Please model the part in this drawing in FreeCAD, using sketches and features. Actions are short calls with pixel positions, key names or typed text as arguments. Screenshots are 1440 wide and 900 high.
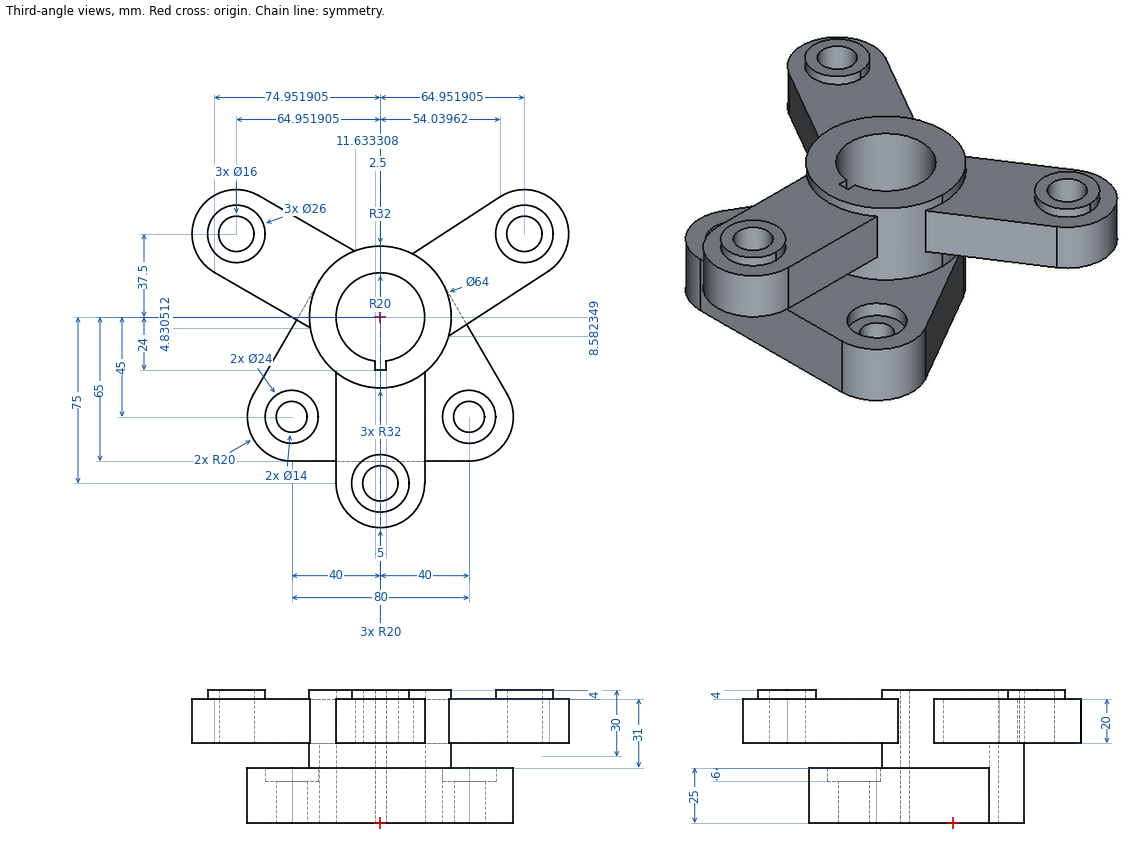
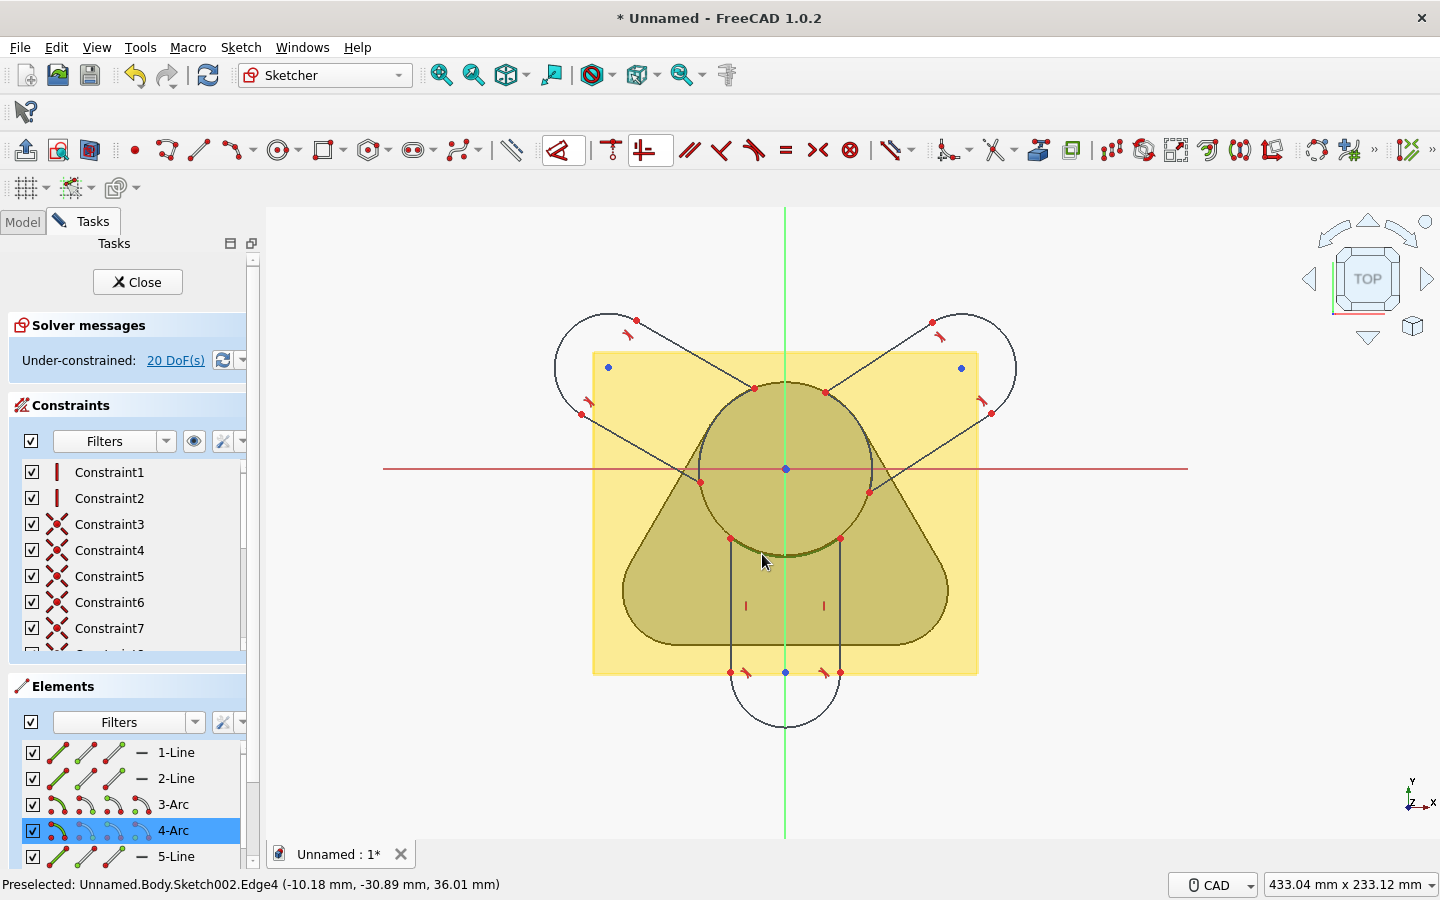
scroll(871, 458, up, 2)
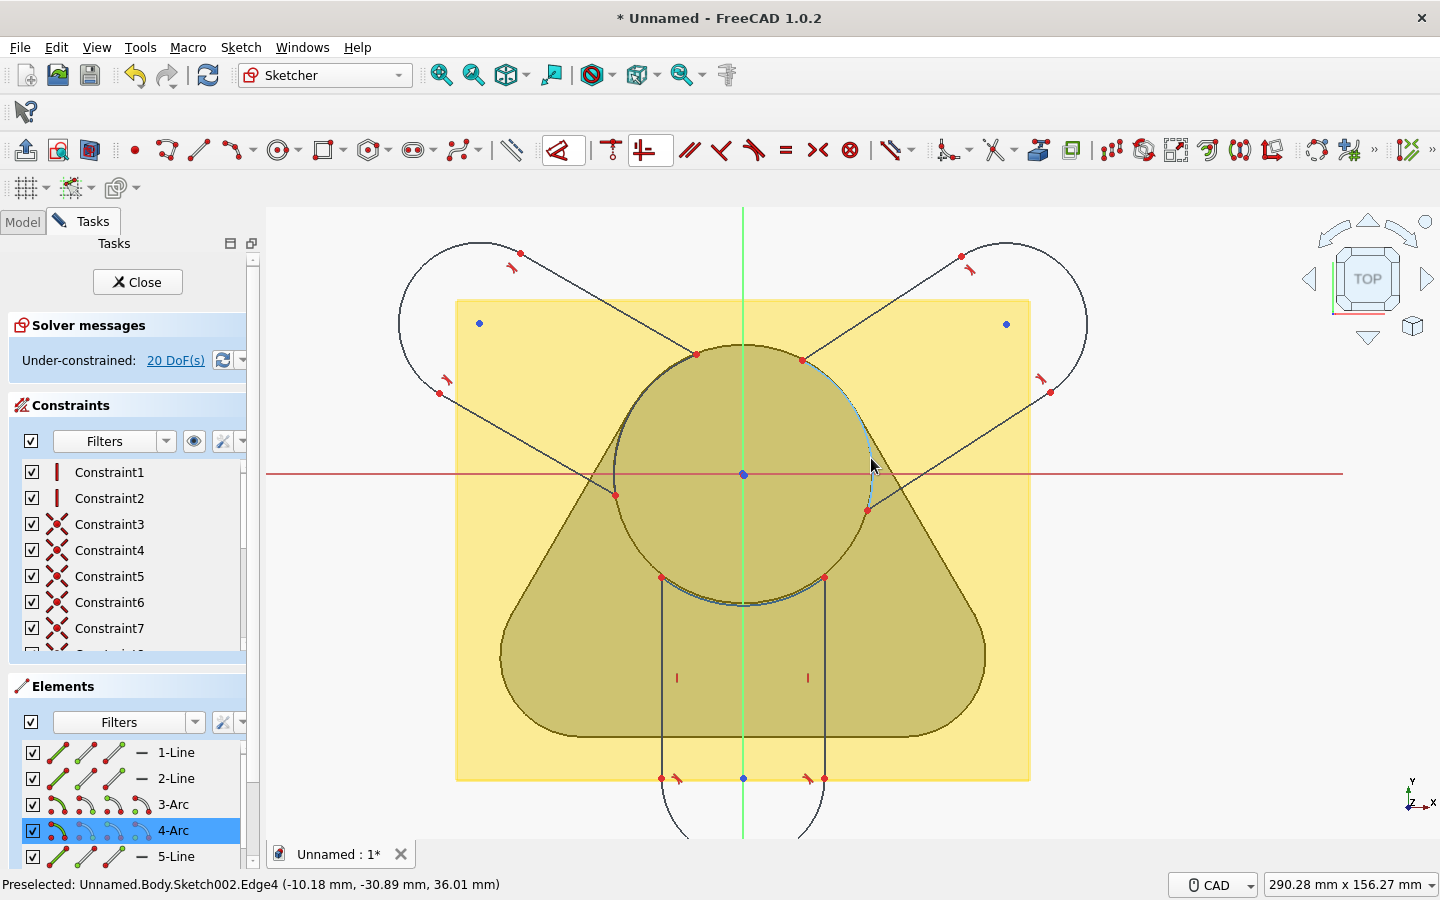
click(871, 457)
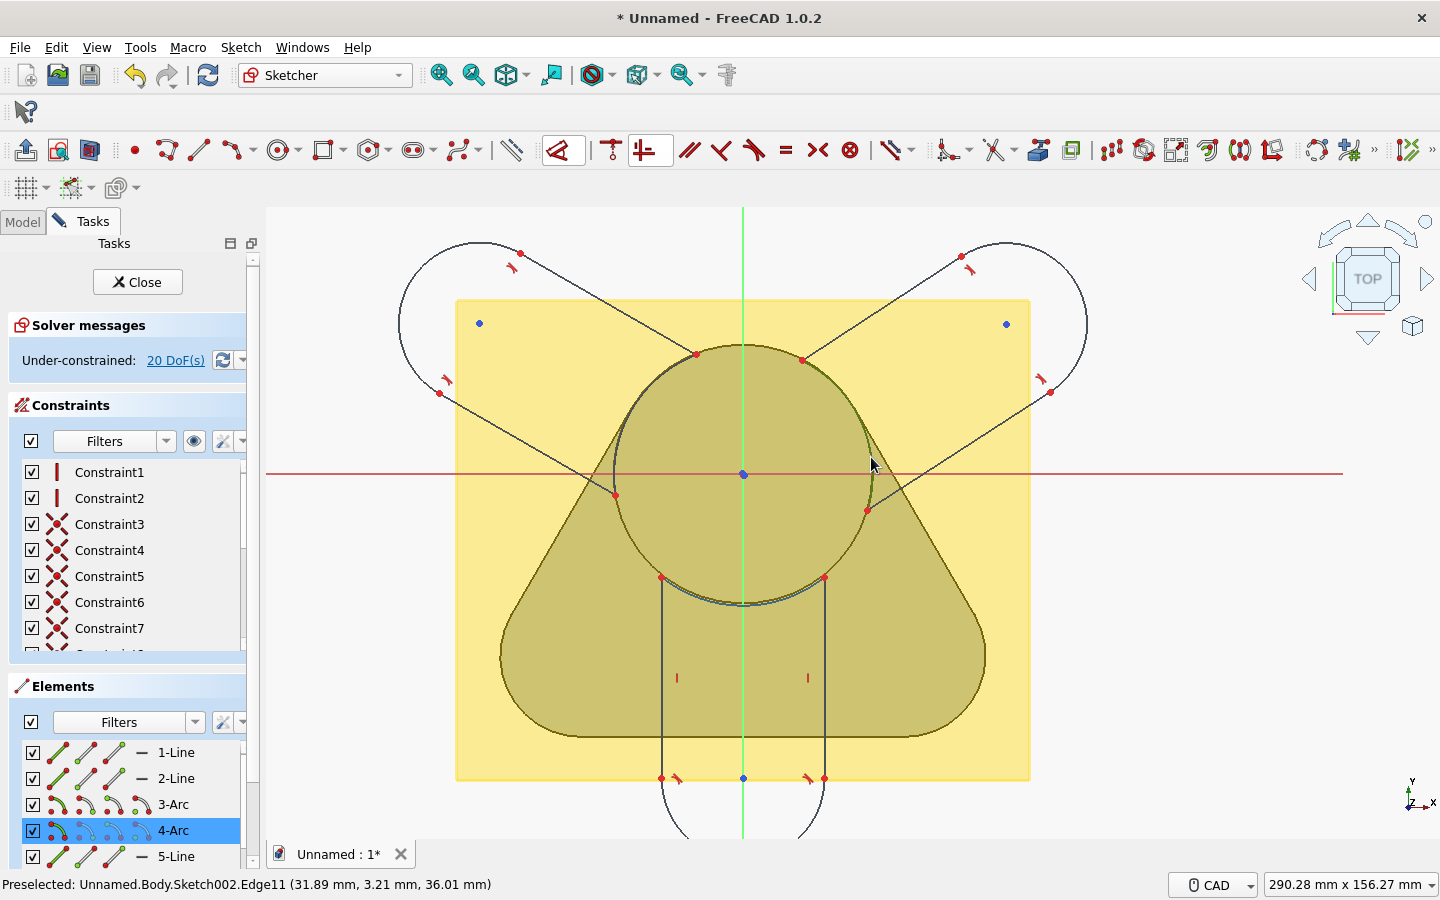
key(c)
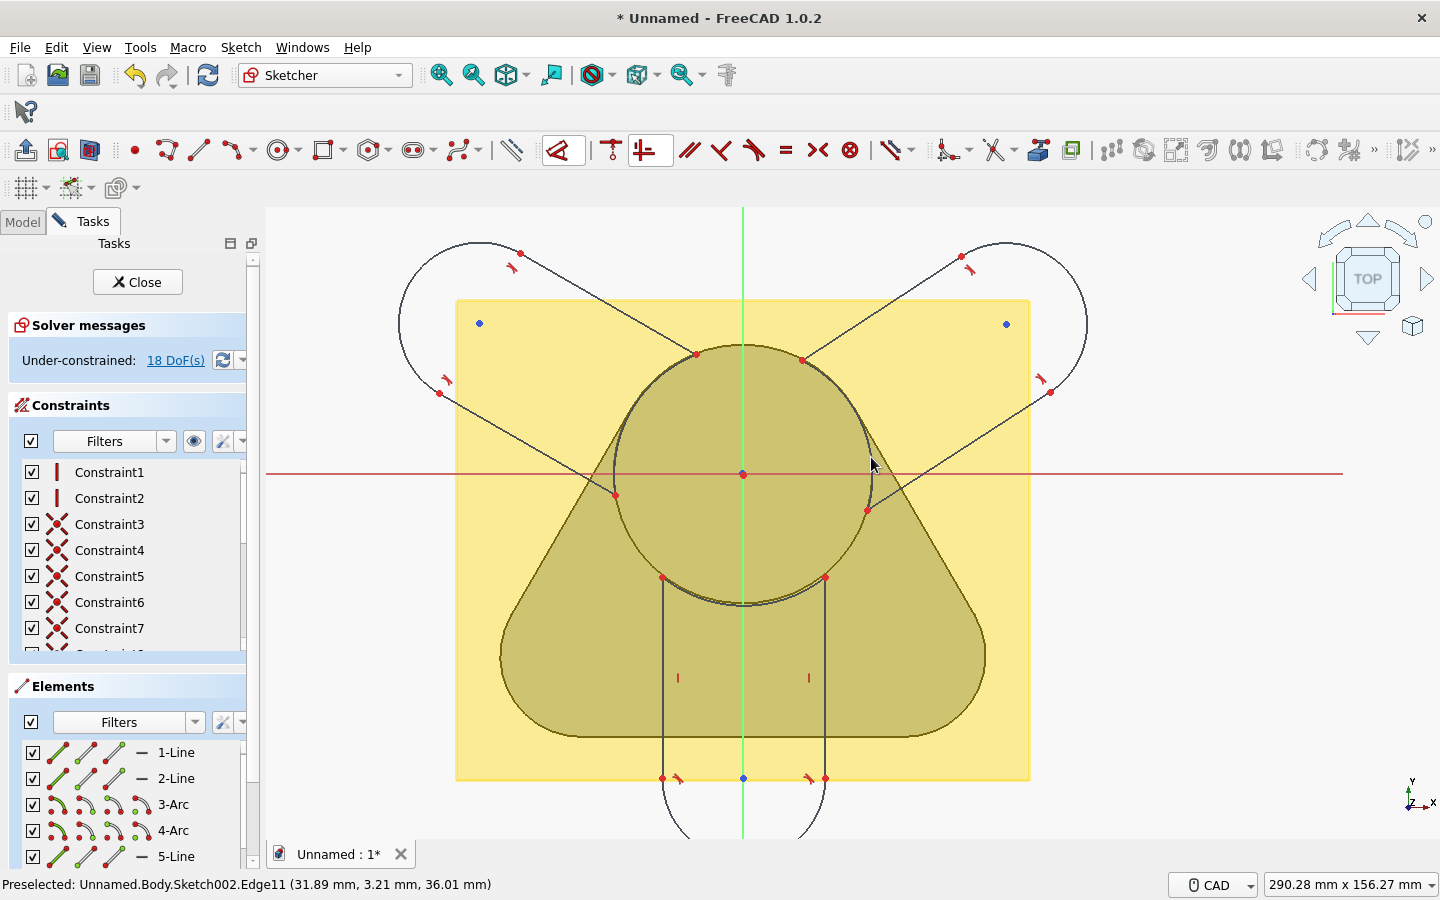
drag(733, 464, 754, 485)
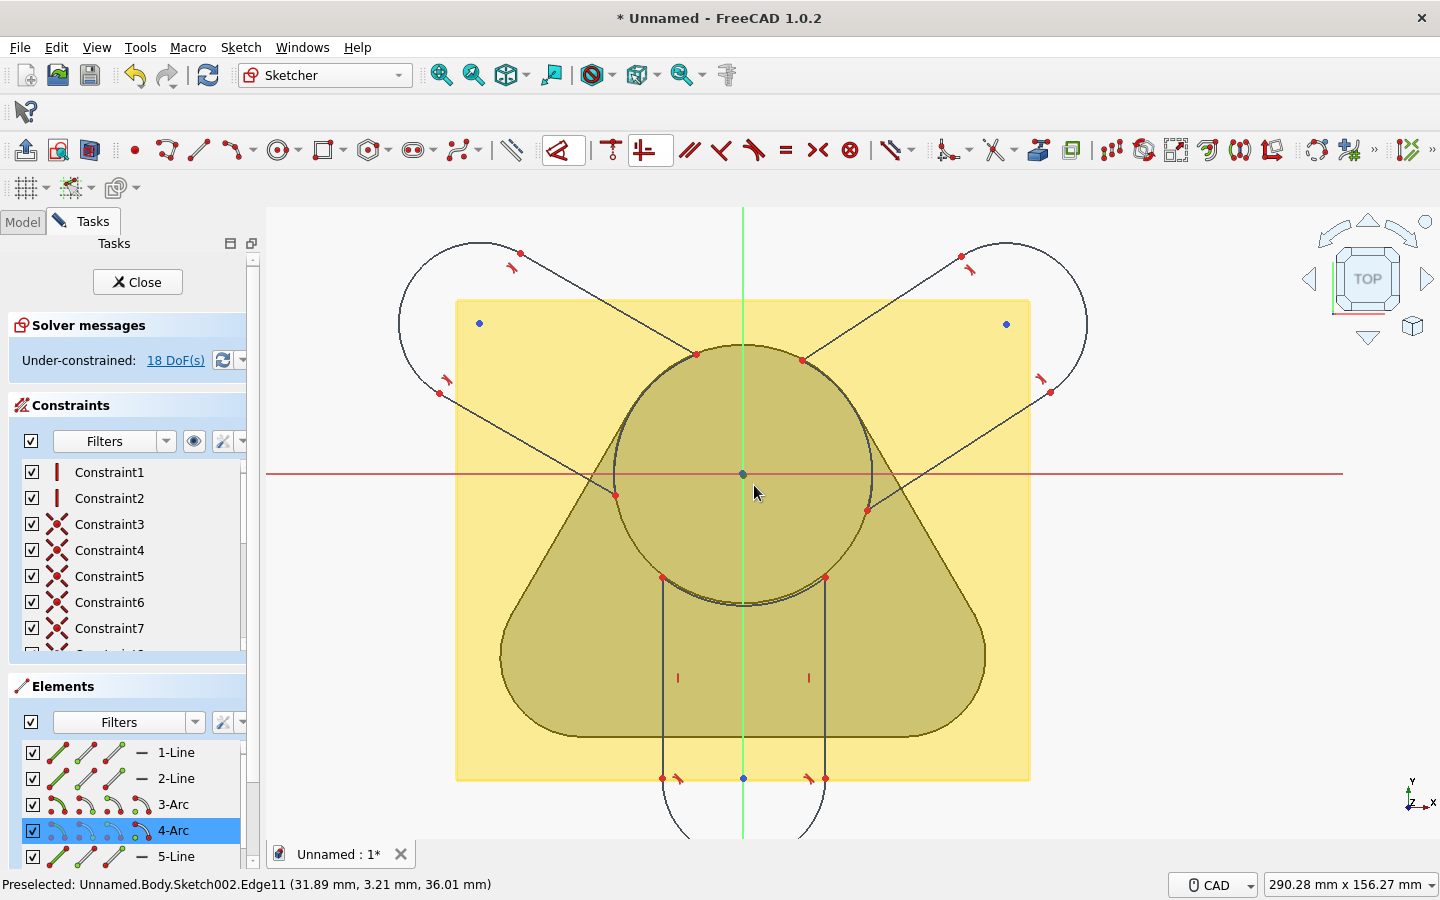
click(612, 150)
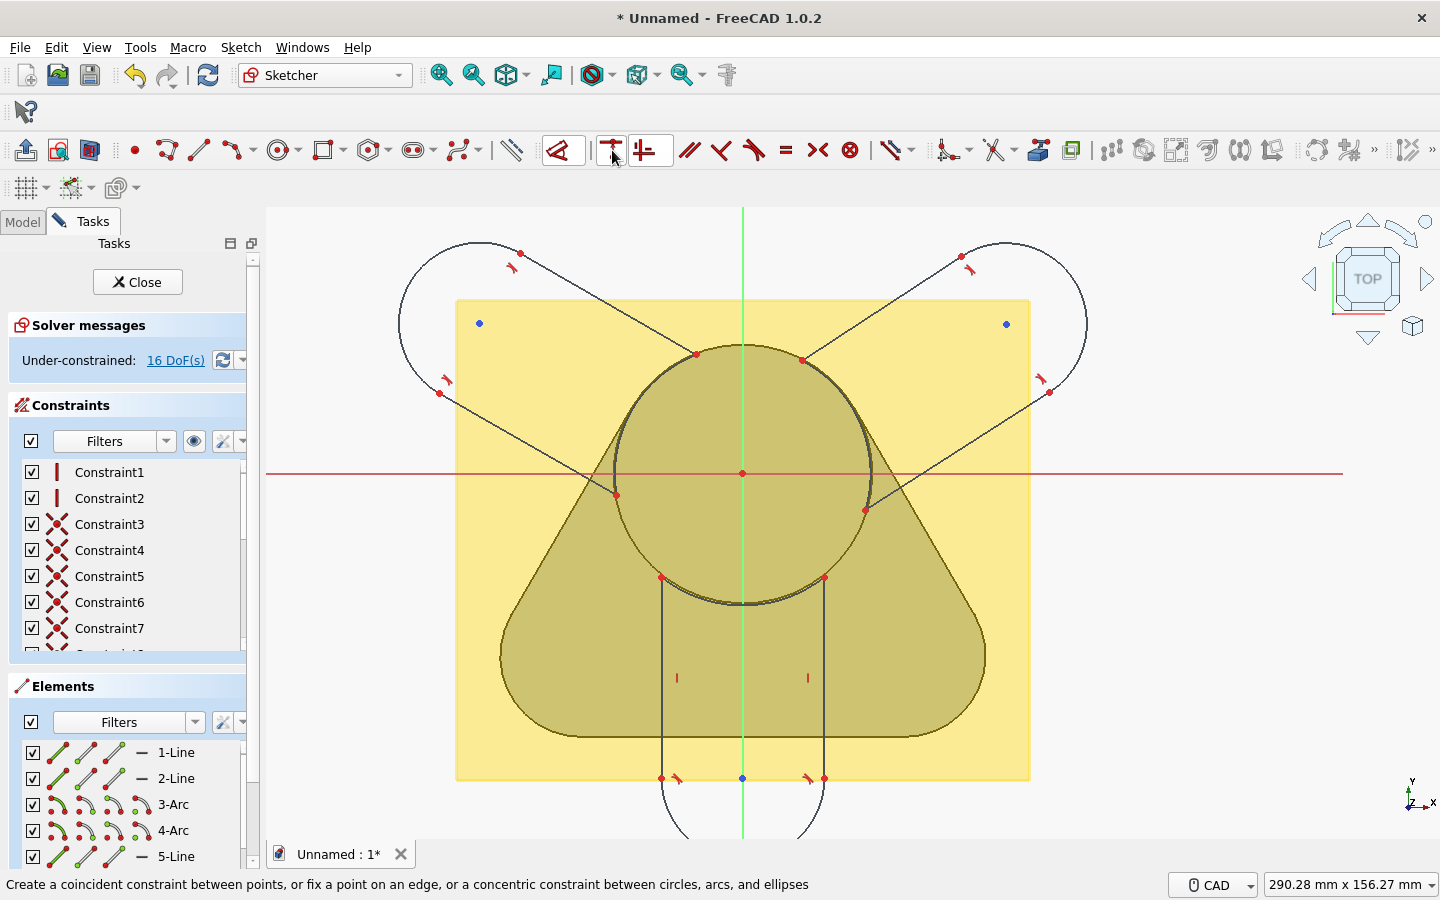
click(708, 601)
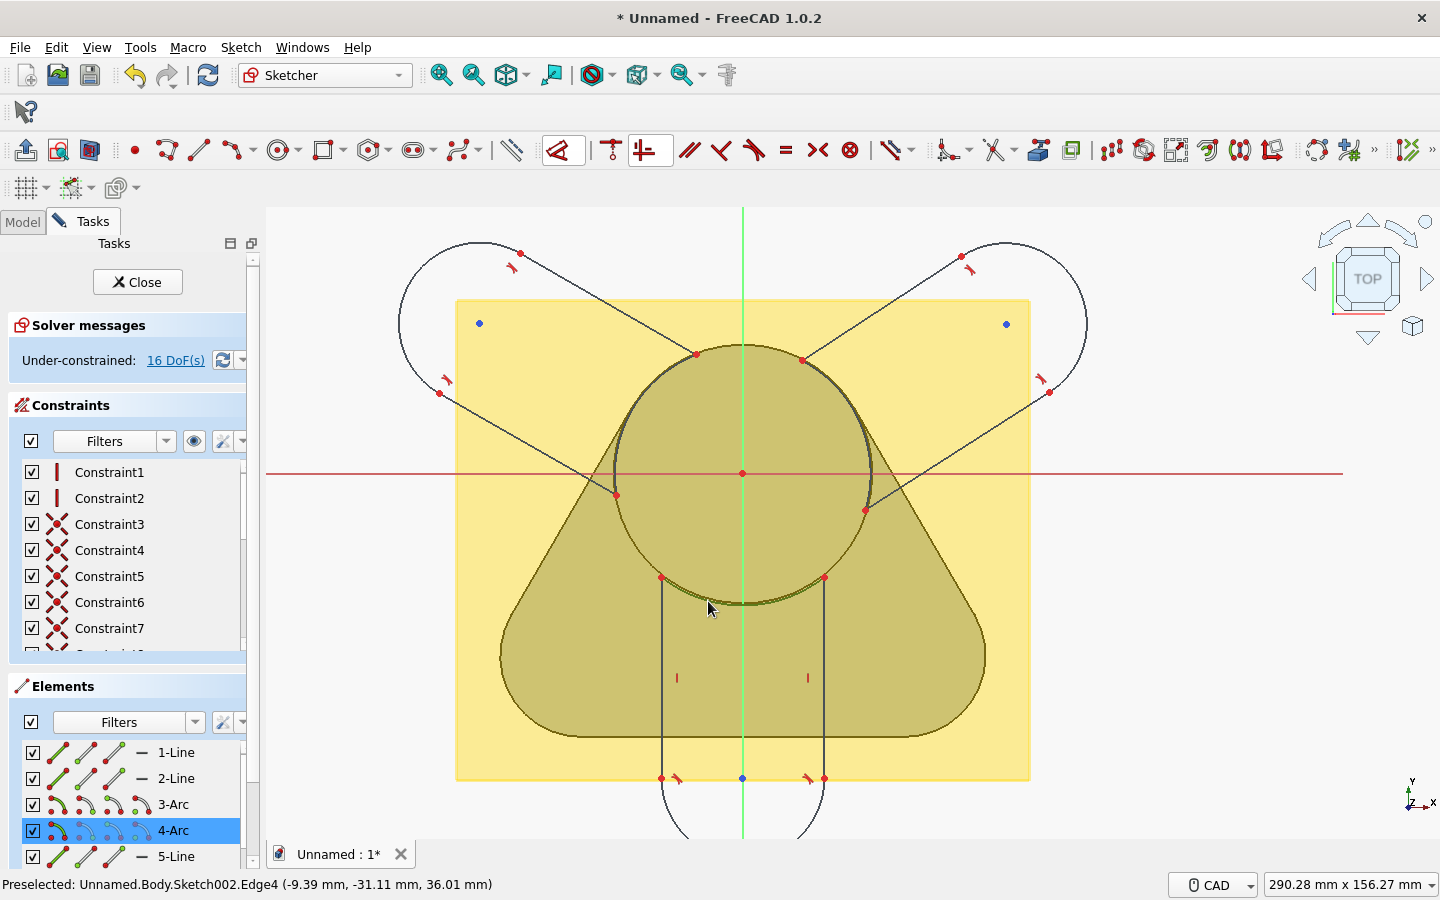
click(653, 383)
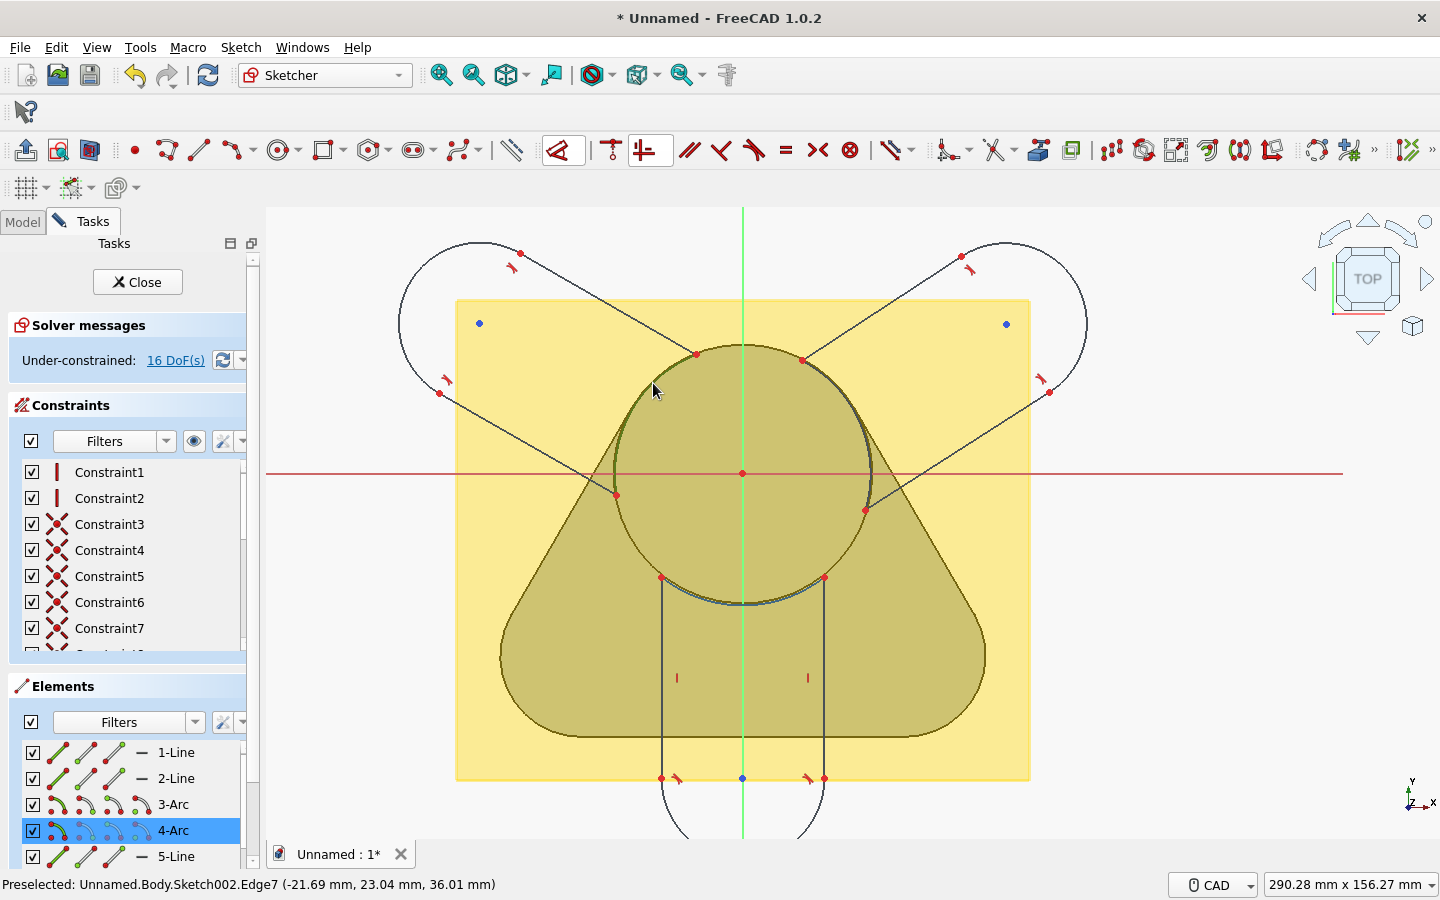
click(870, 458)